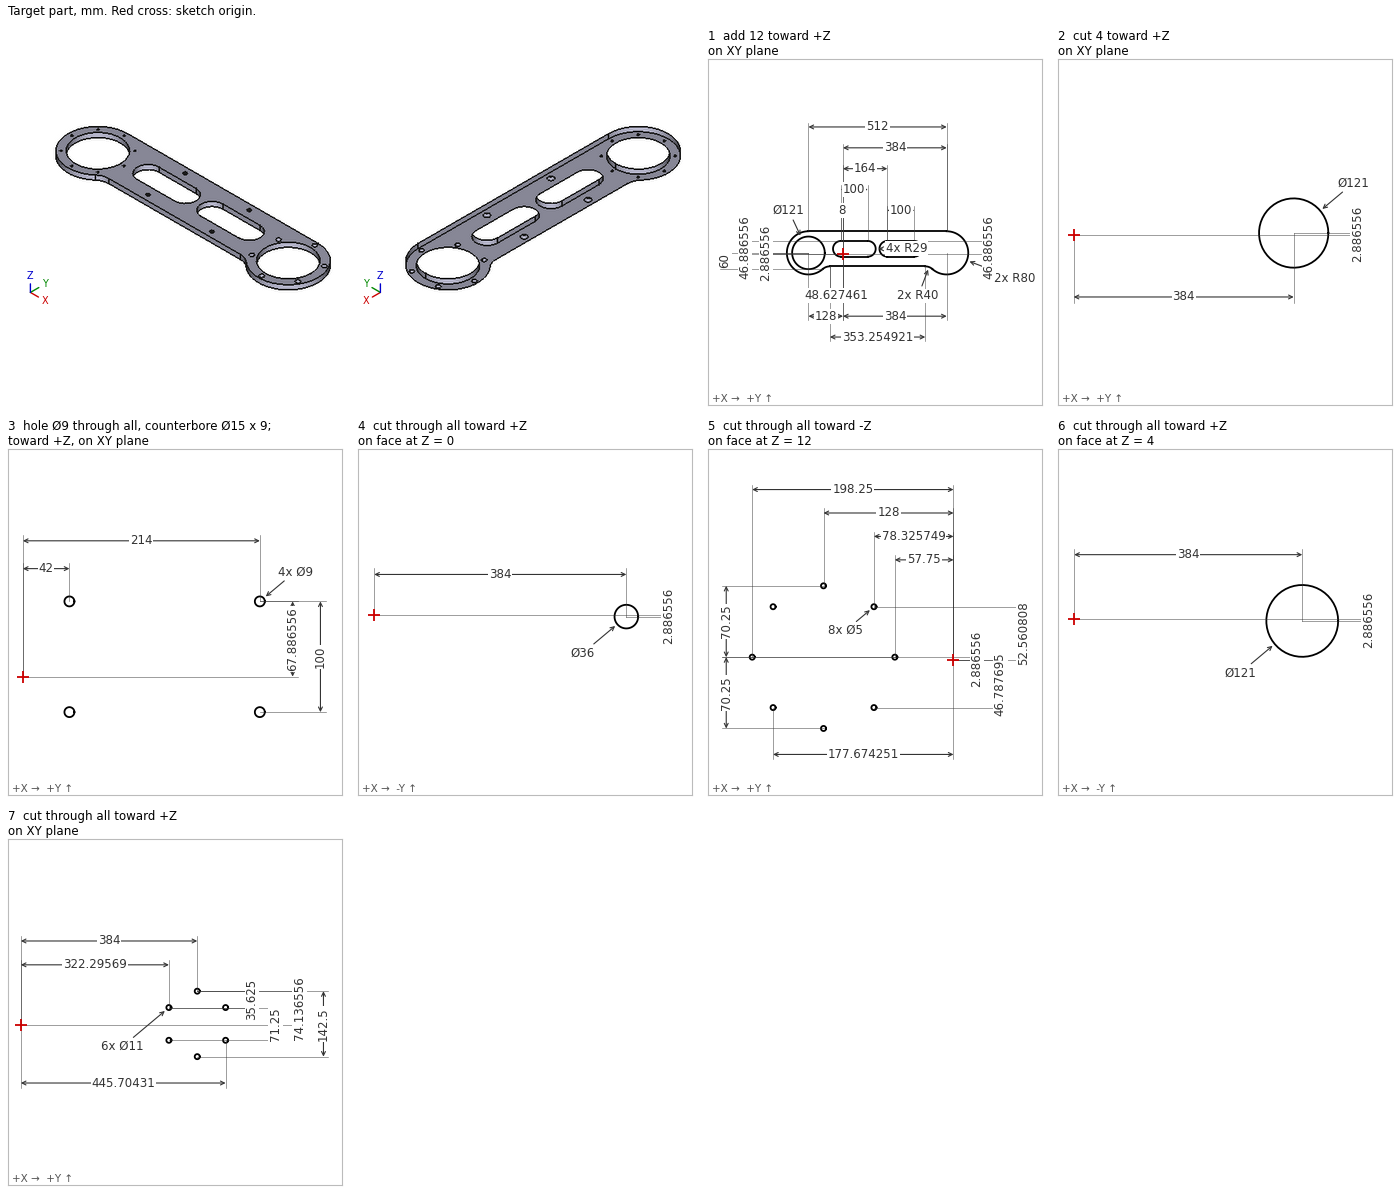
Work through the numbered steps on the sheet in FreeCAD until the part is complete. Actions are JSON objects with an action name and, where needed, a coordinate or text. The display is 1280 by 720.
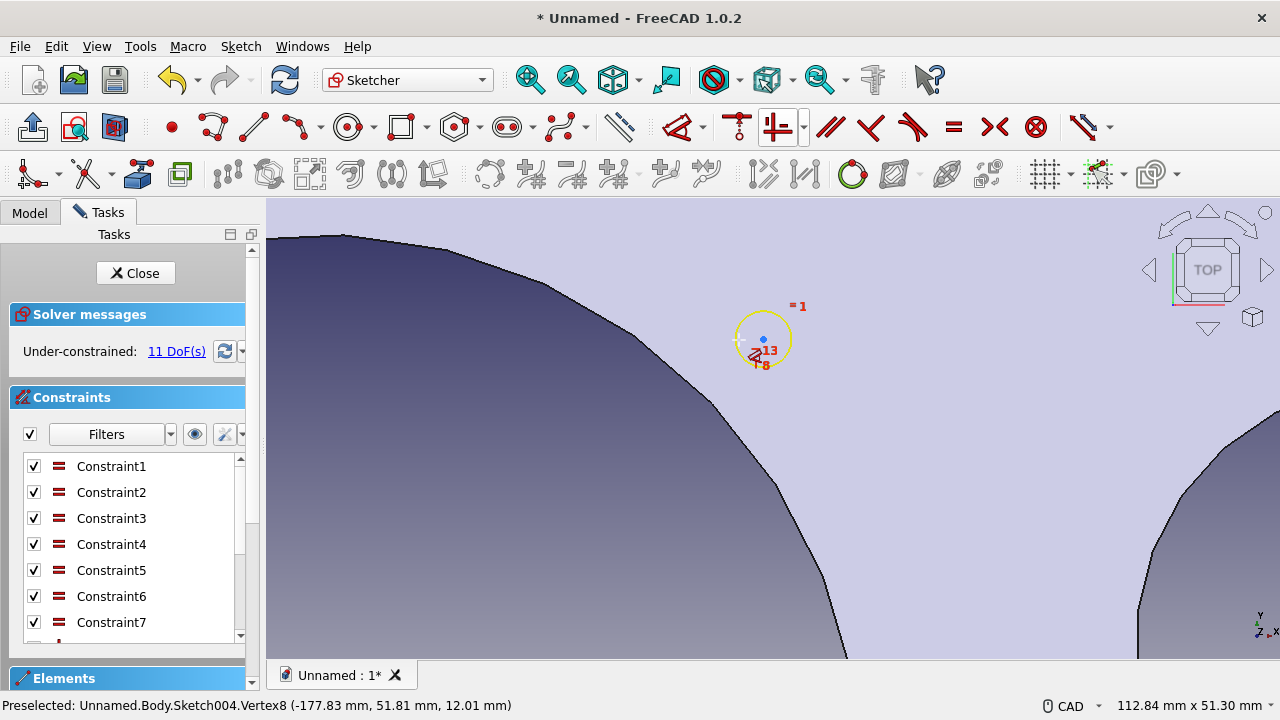
{"action": "left_click", "coordinate": [736, 338]}
{"action": "left_click", "coordinate": [704, 337]}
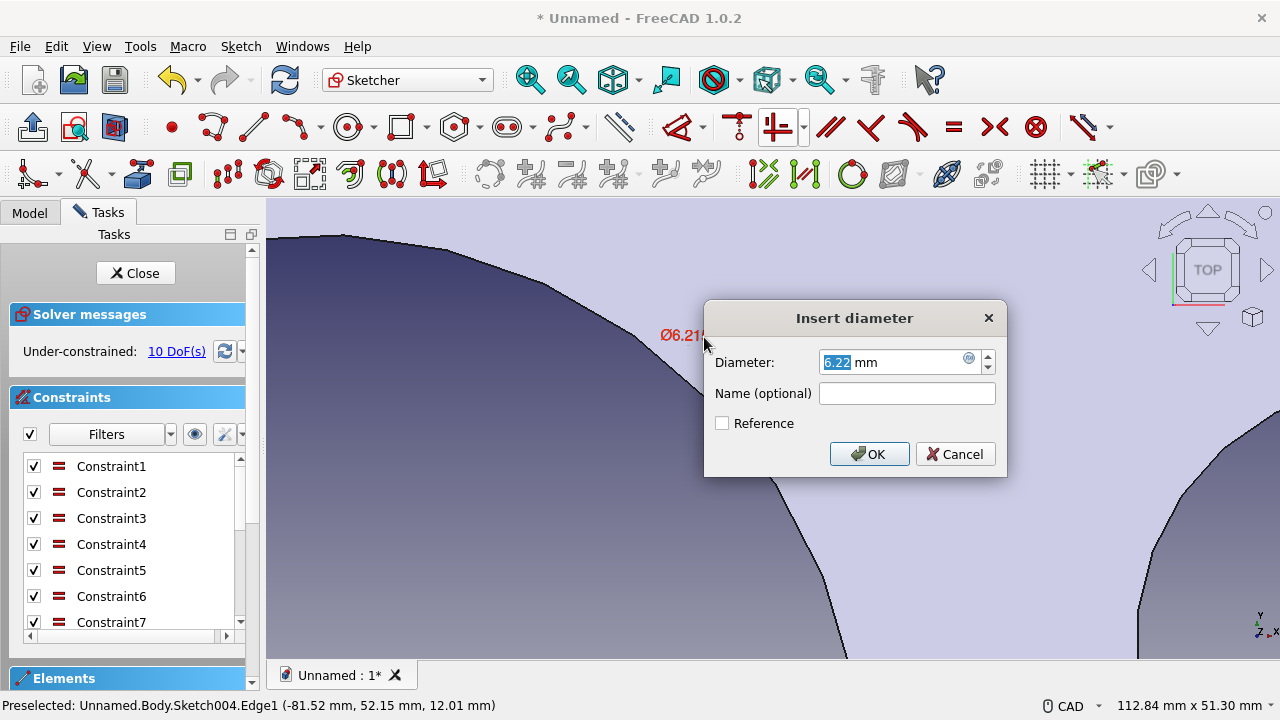
{"action": "type", "text": "5"}
{"action": "key", "text": "Return"}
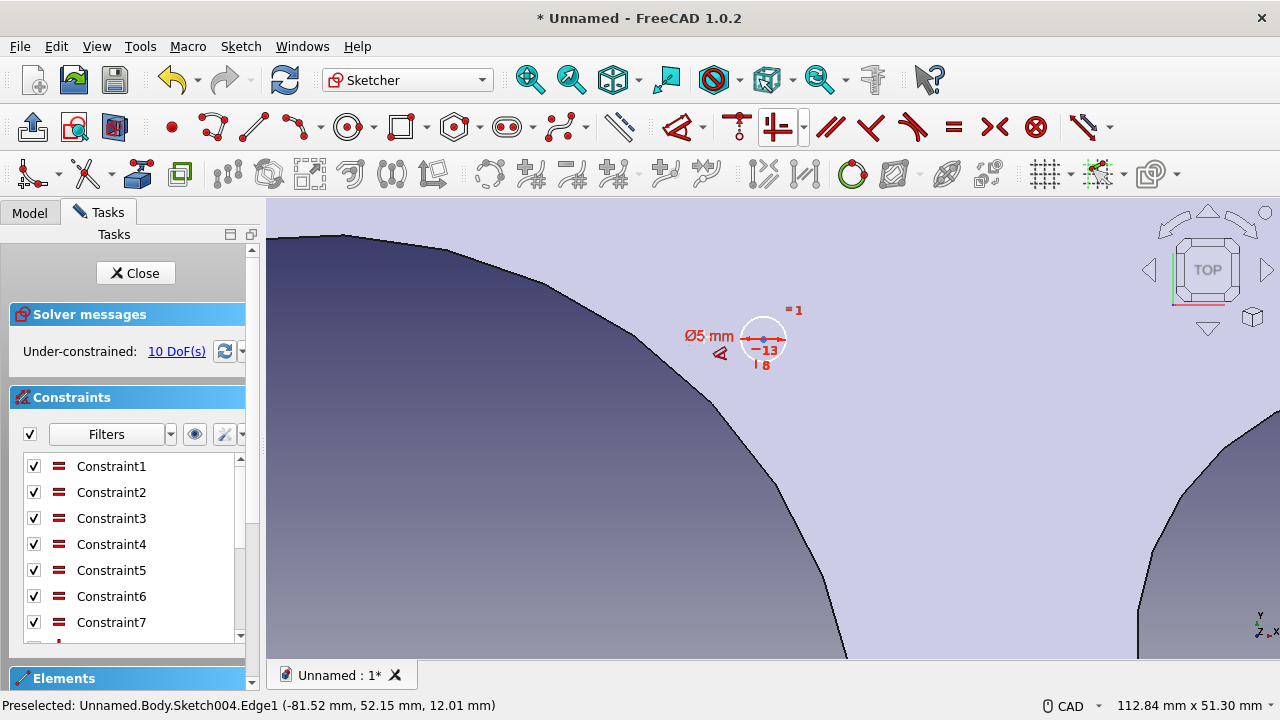
{"action": "scroll", "coordinate": [739, 340], "scroll_direction": "down", "scroll_amount": 8}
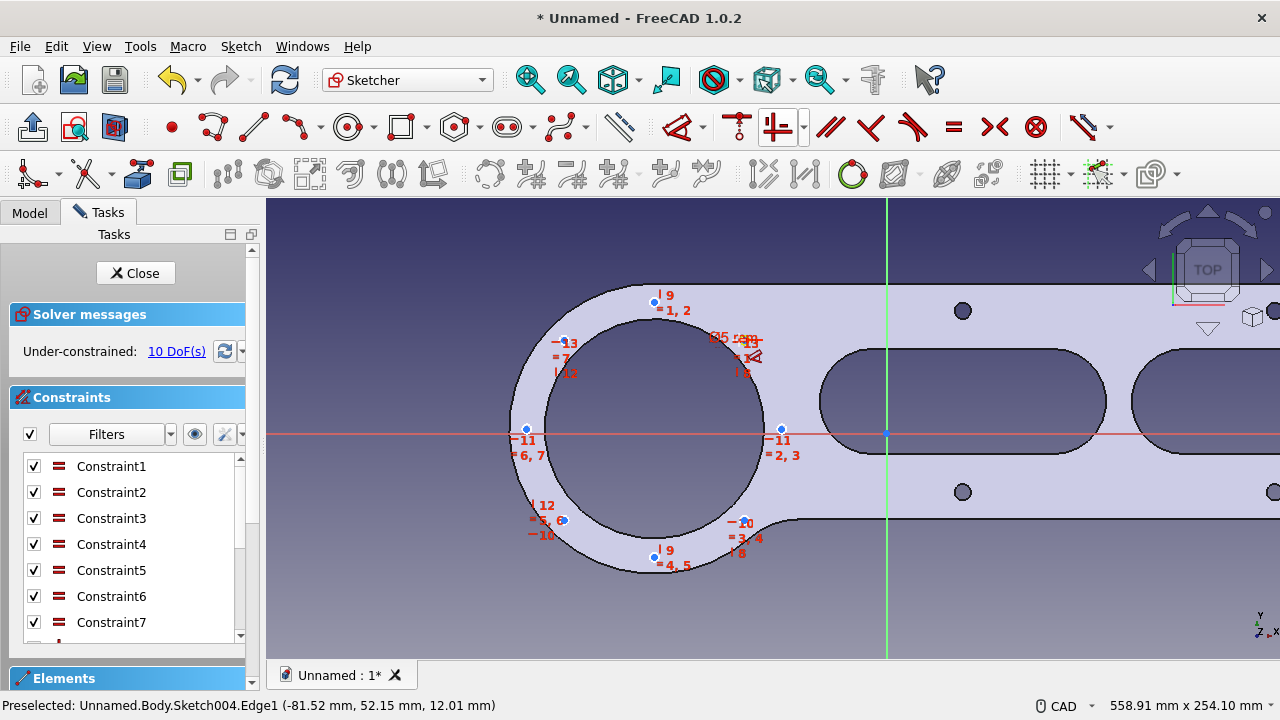
{"action": "left_click", "coordinate": [654, 302]}
{"action": "left_click", "coordinate": [770, 268]}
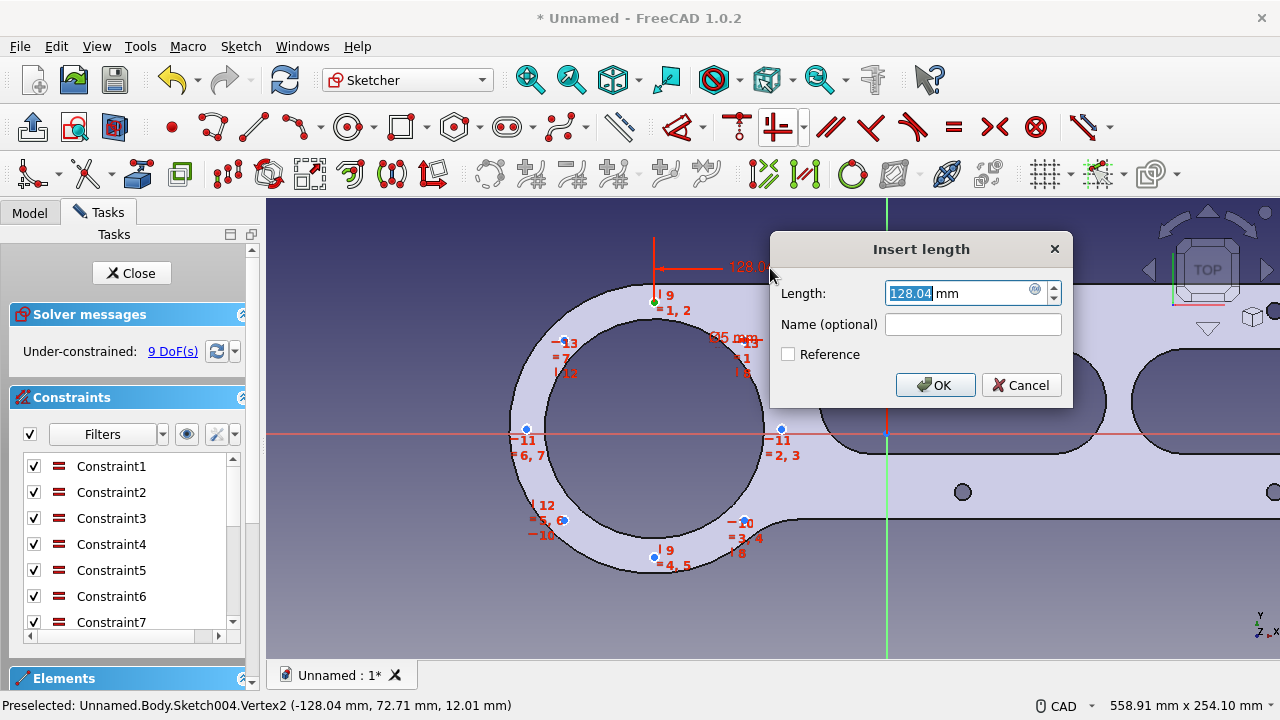
{"action": "type", "text": "128"}
{"action": "key", "text": "Return"}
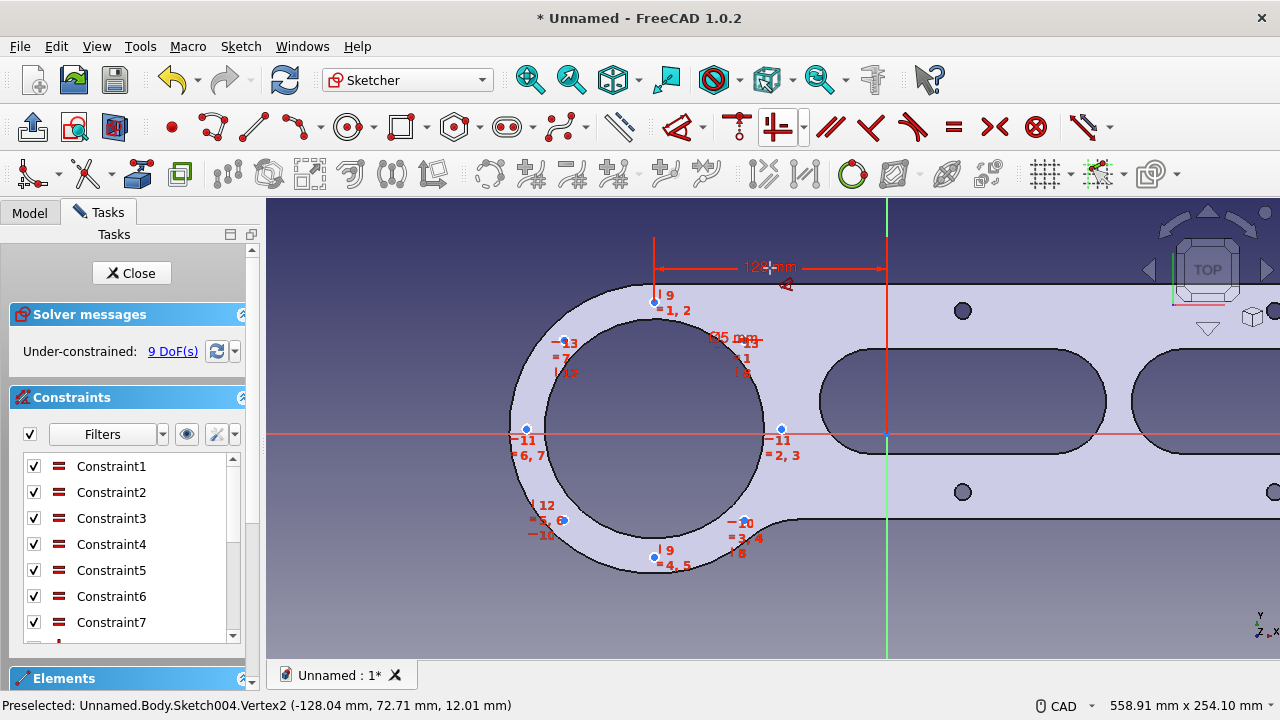
{"action": "left_click", "coordinate": [782, 429]}
{"action": "left_click", "coordinate": [834, 468]}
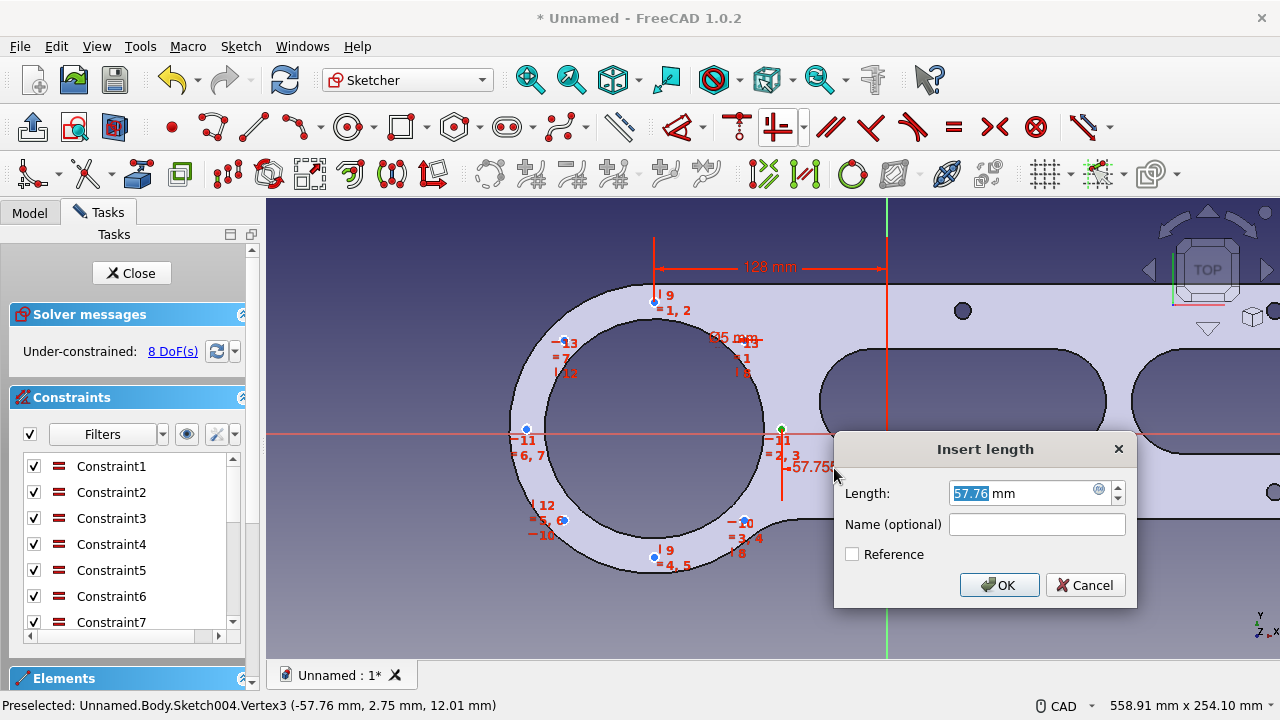
{"action": "type", "text": "57.75"}
{"action": "key", "text": "Return"}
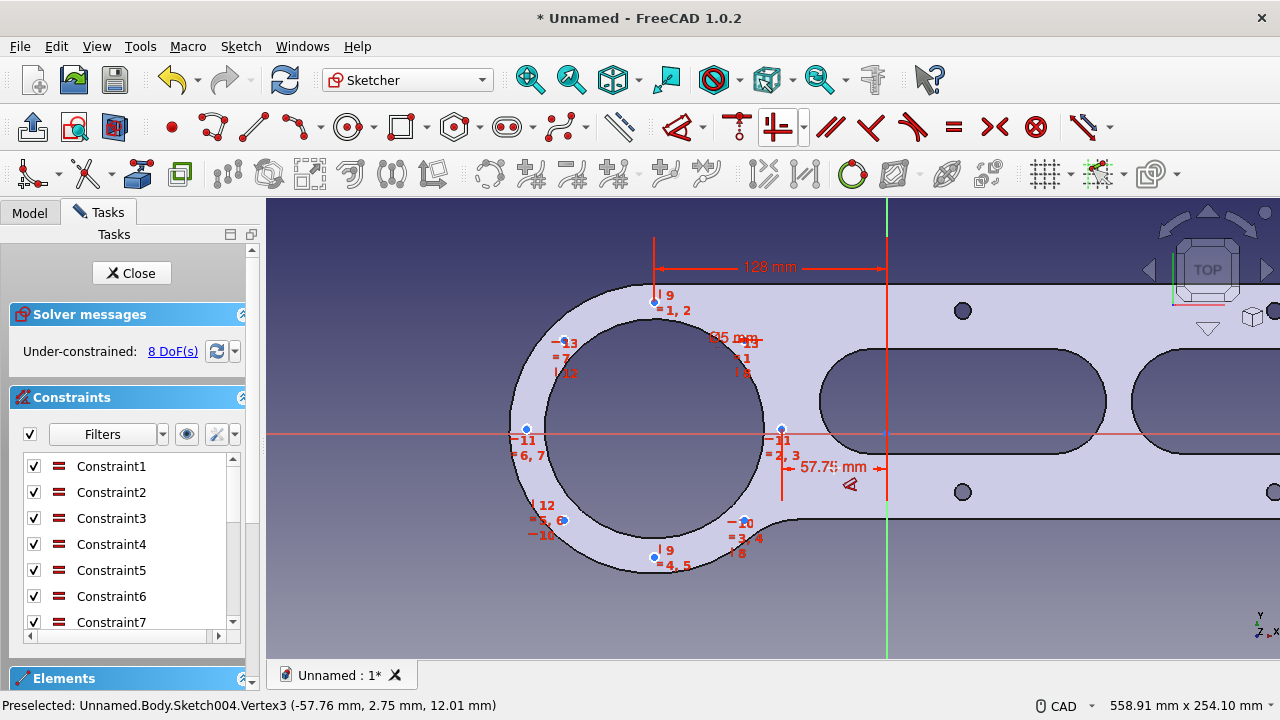
{"action": "left_click", "coordinate": [527, 429]}
{"action": "left_click", "coordinate": [707, 468]}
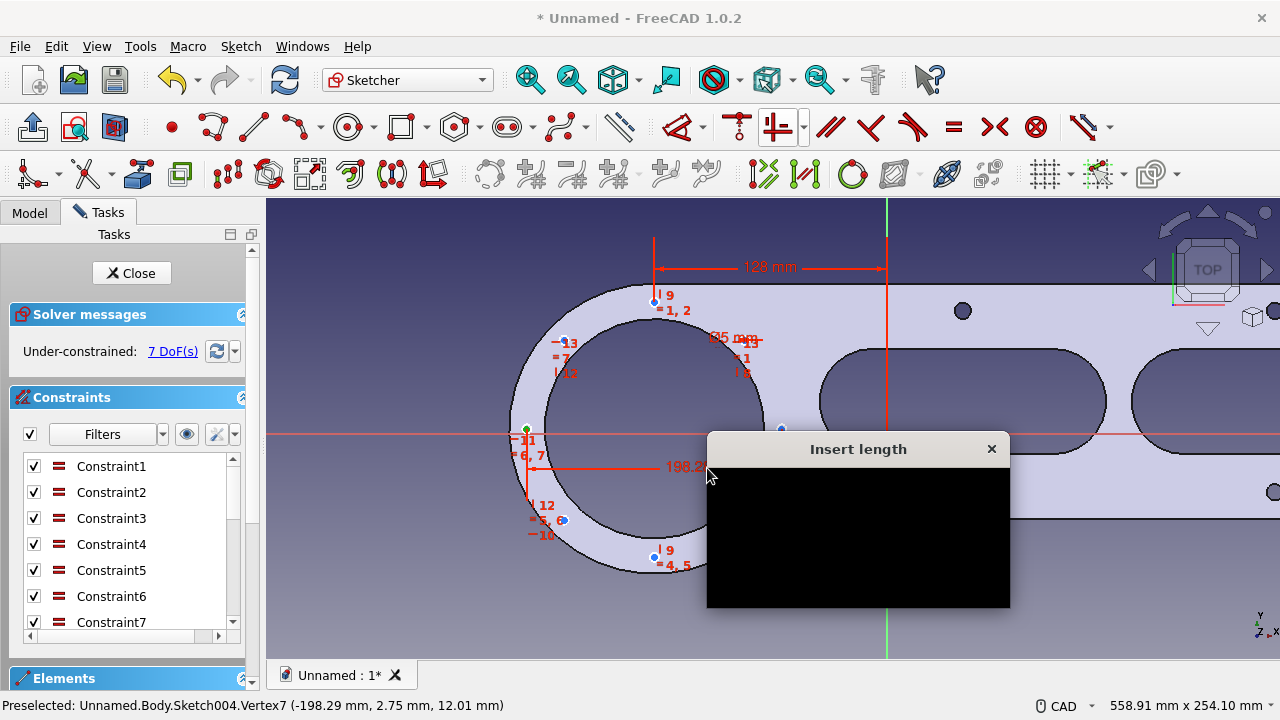
{"action": "type", "text": "198.25"}
{"action": "key", "text": "Return"}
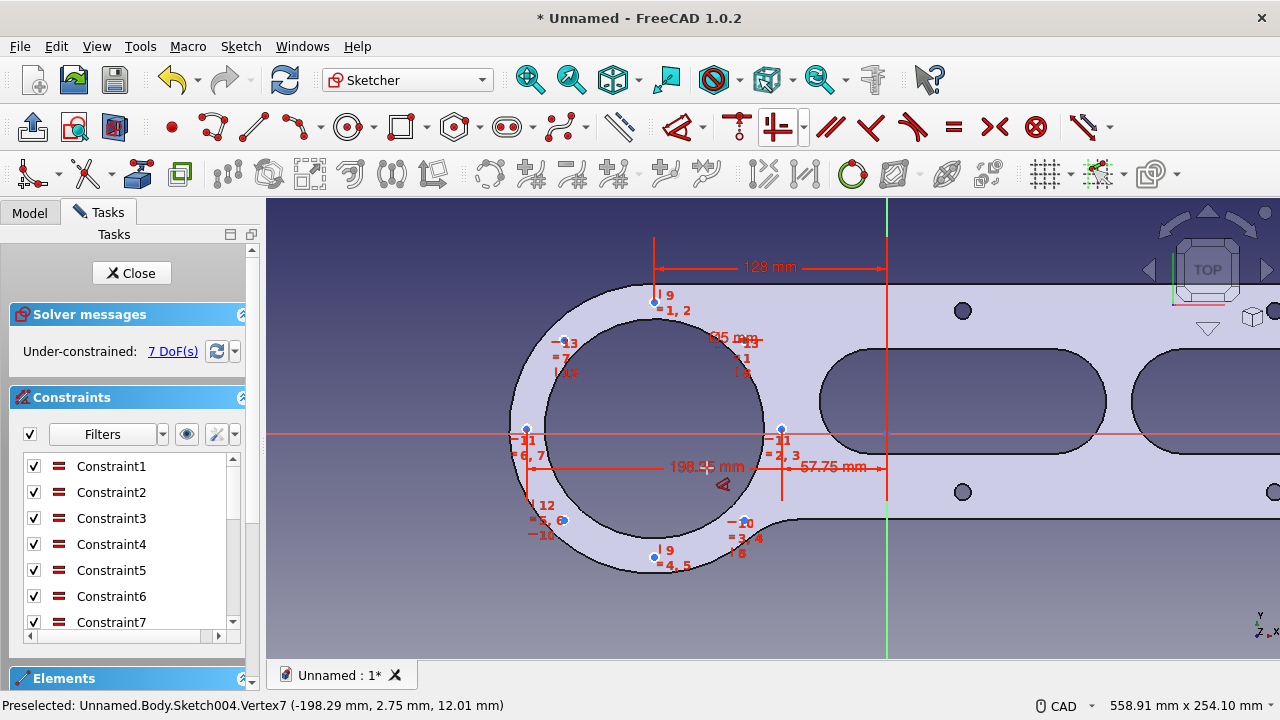
{"action": "left_click", "coordinate": [654, 302]}